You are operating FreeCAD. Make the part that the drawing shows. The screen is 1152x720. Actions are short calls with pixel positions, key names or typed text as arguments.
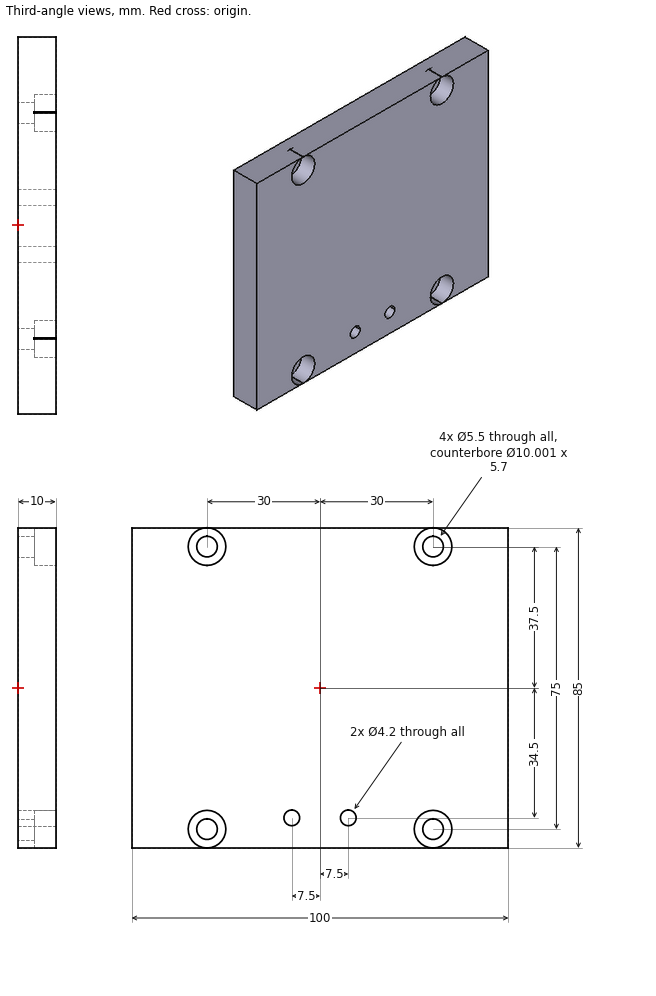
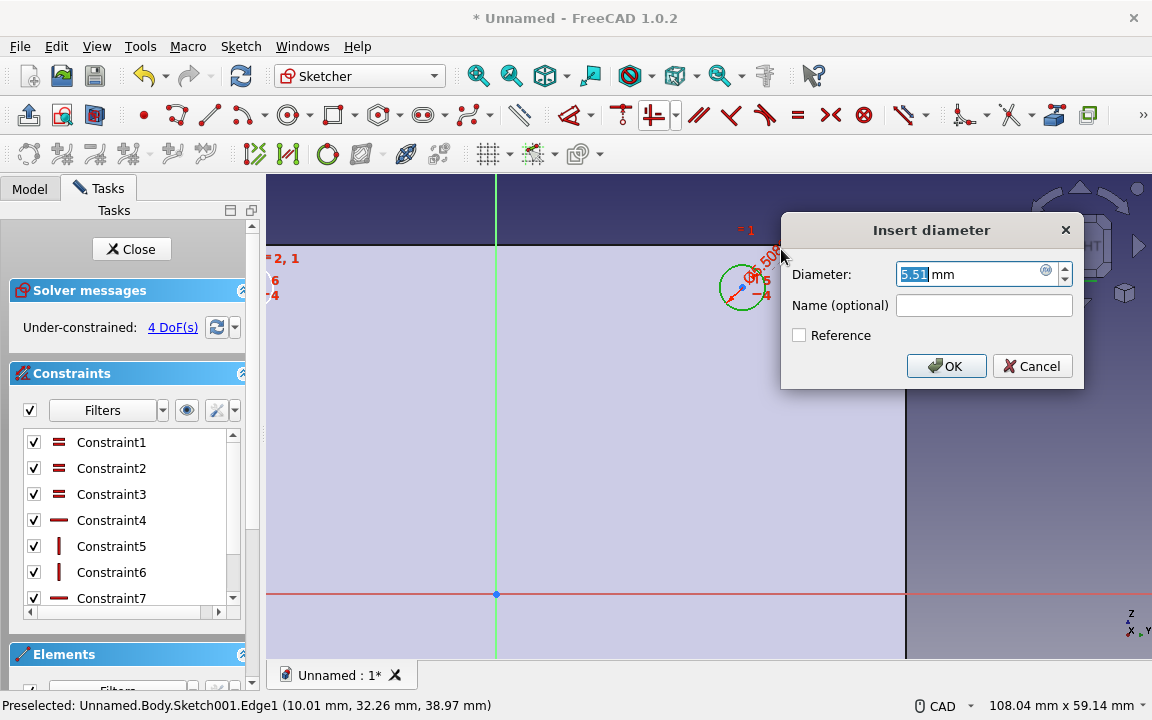
text(5.5)
key(Return)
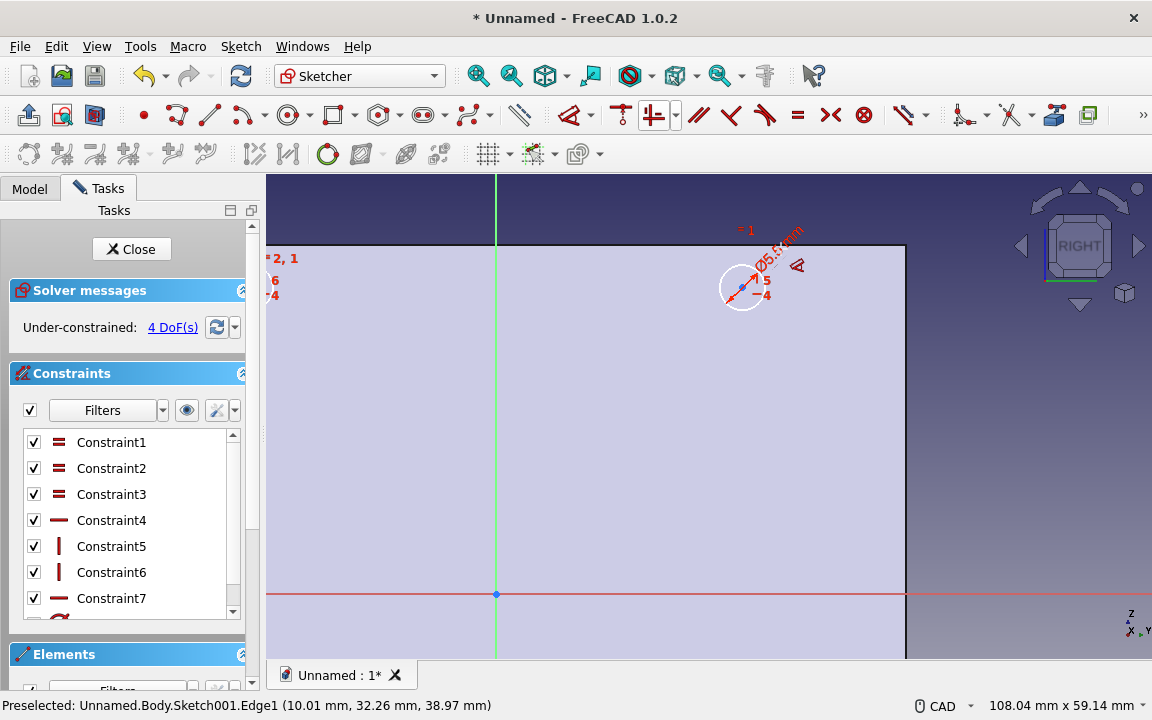
click(742, 288)
click(619, 254)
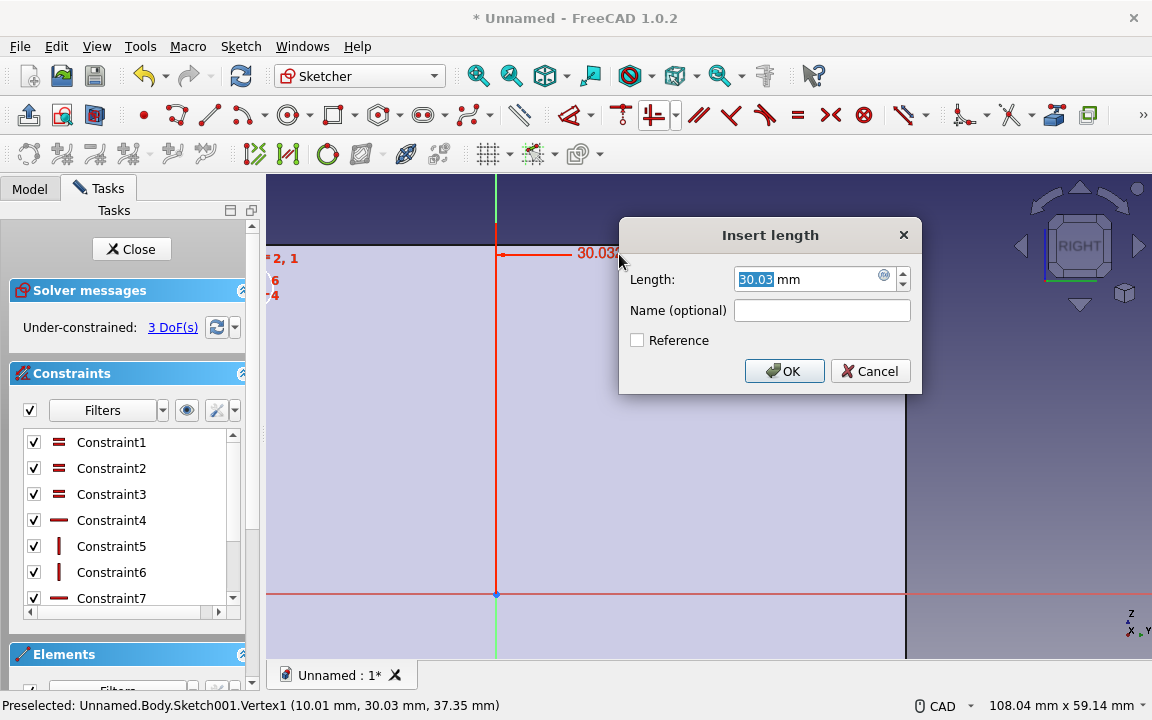
text(30)
key(Return)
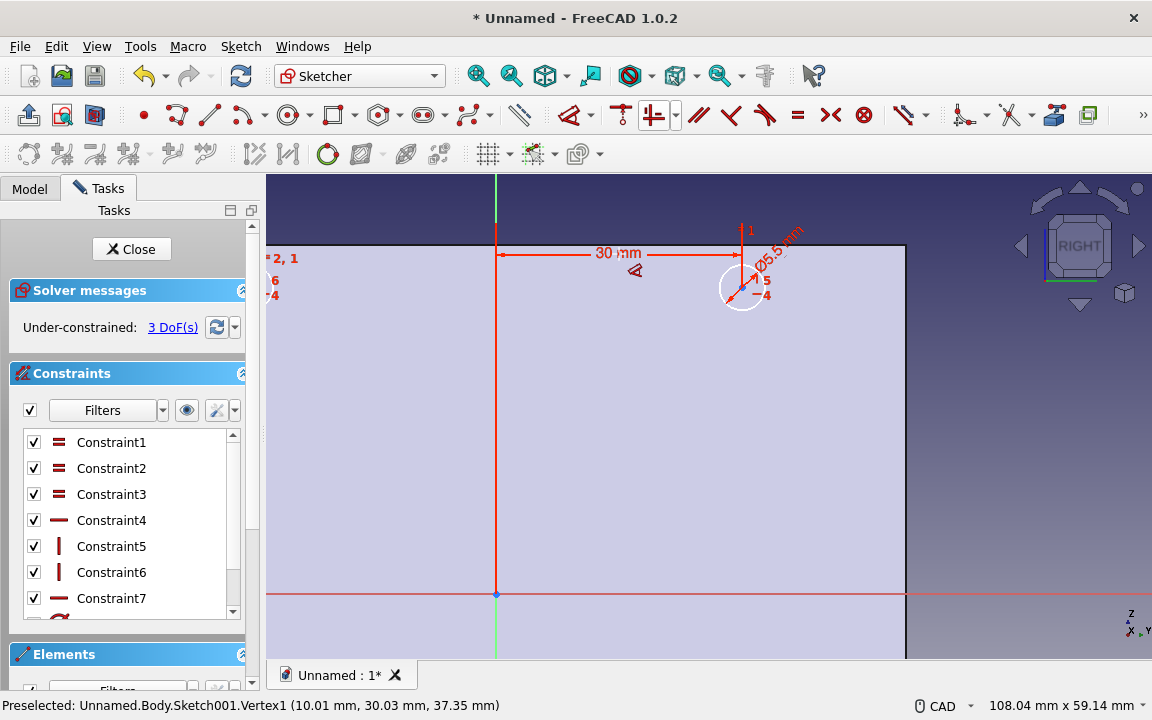
scroll(758, 272, down, 4)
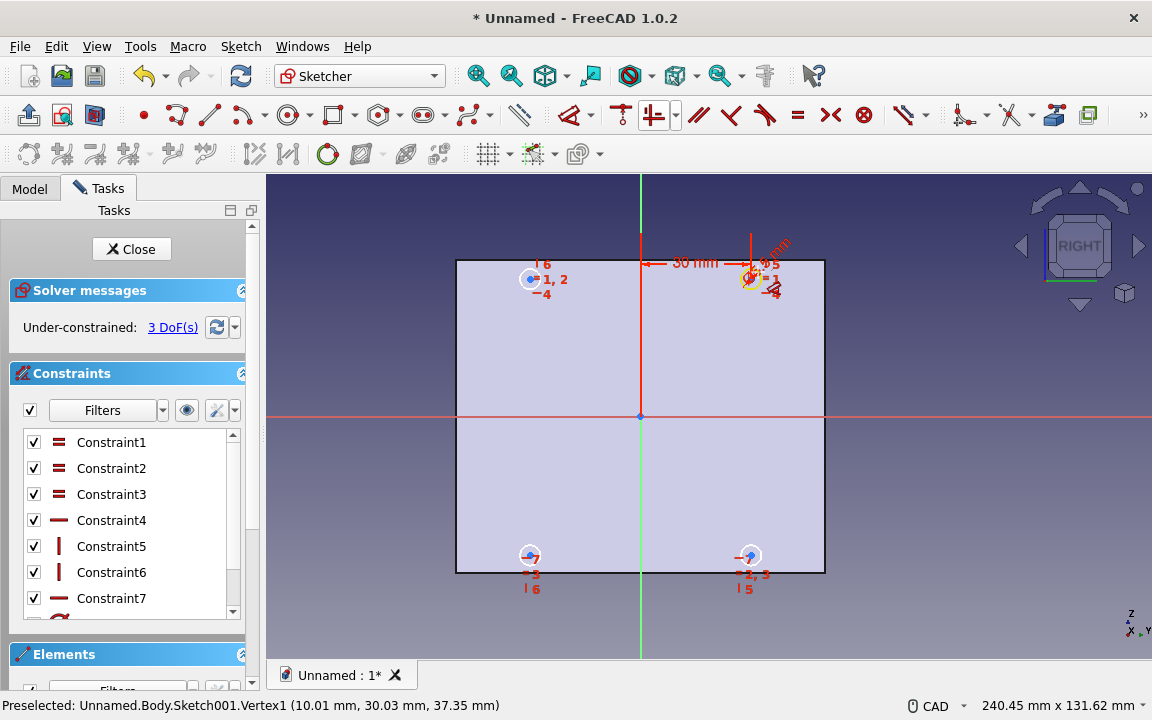
click(530, 279)
click(585, 245)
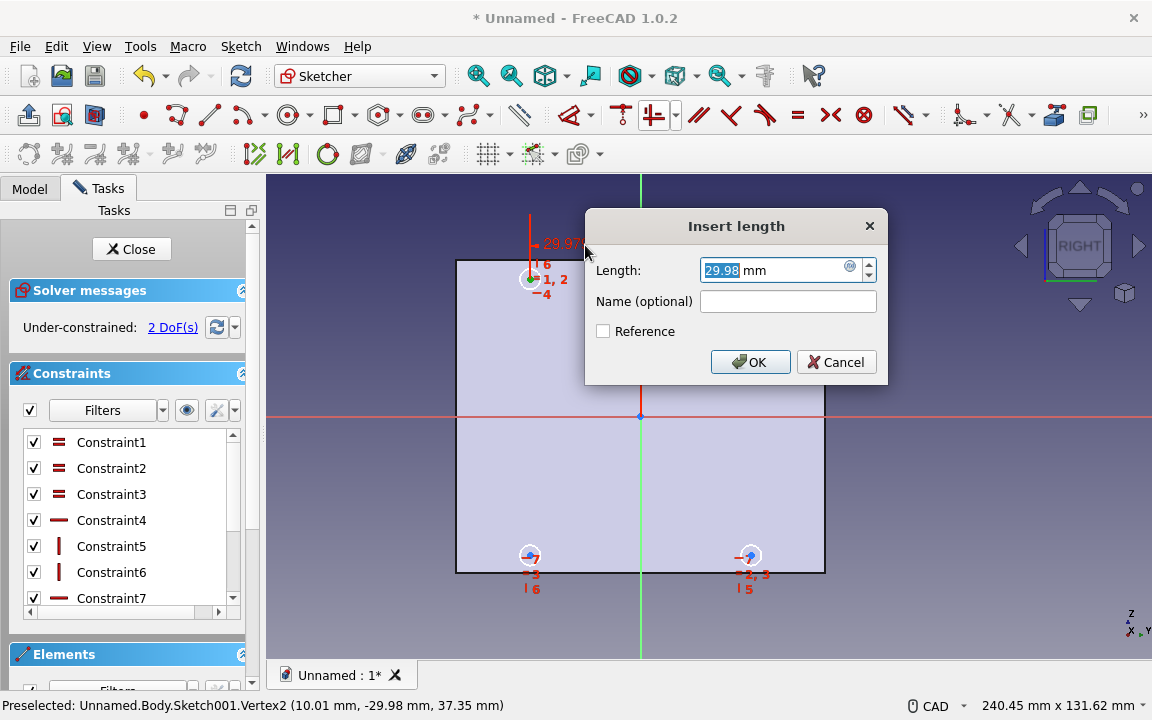
text(30)
key(Return)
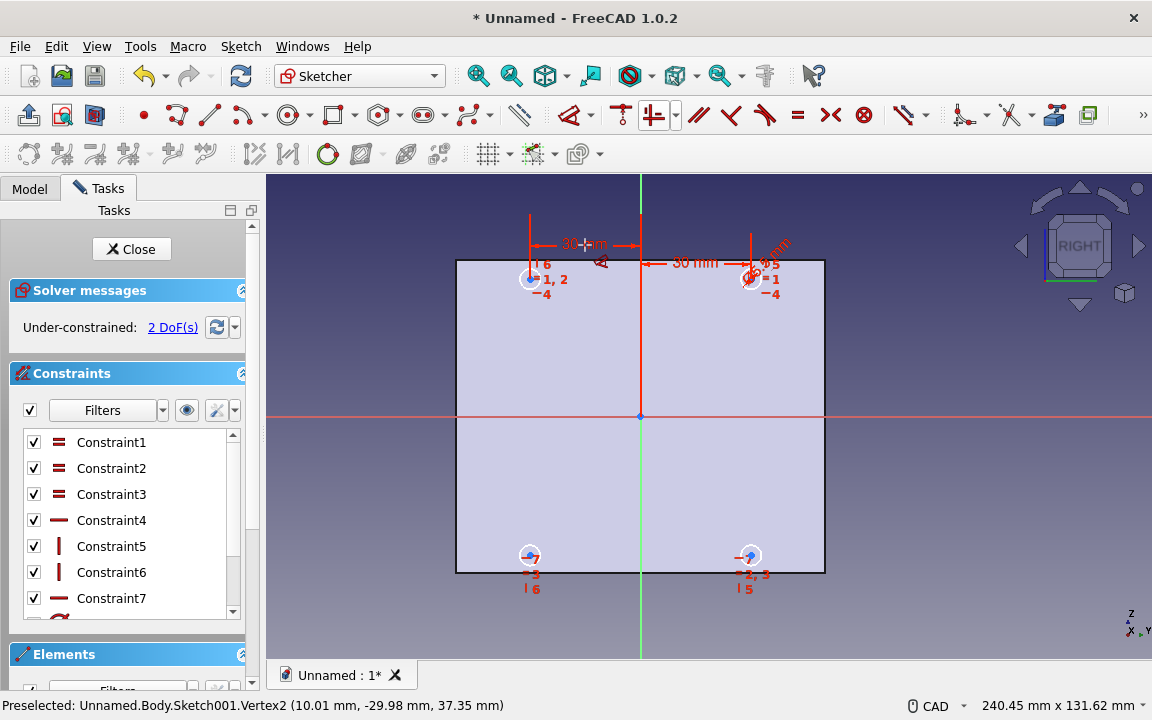
click(751, 279)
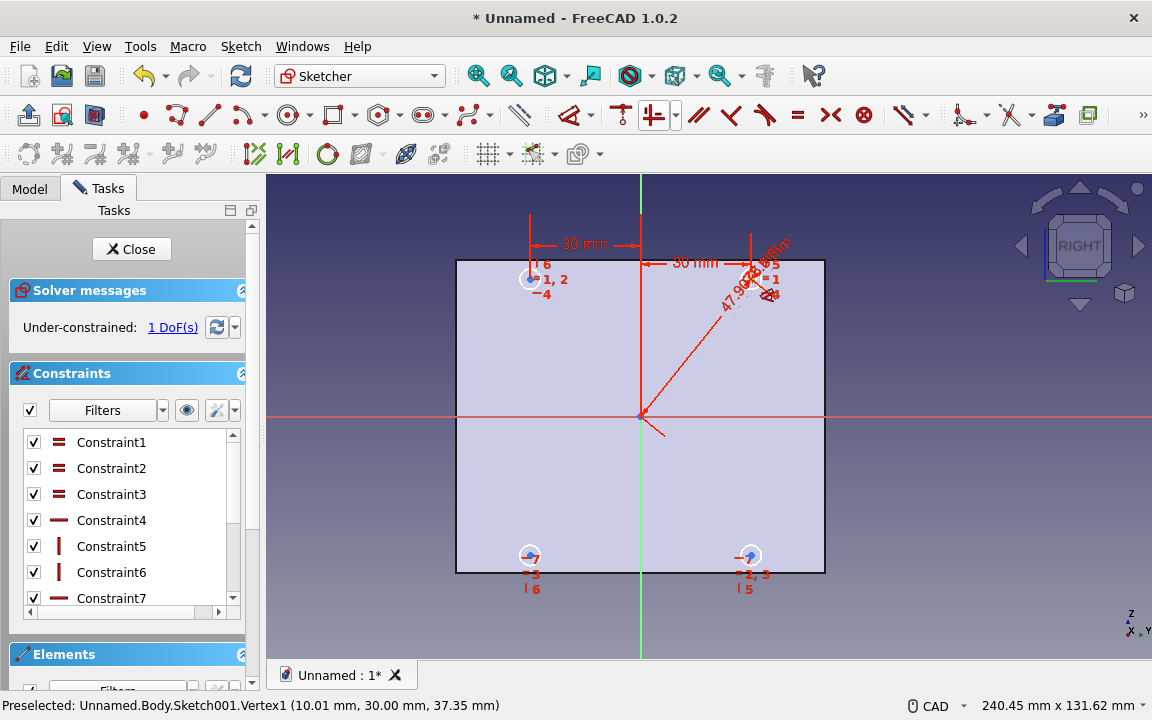
click(751, 555)
click(785, 354)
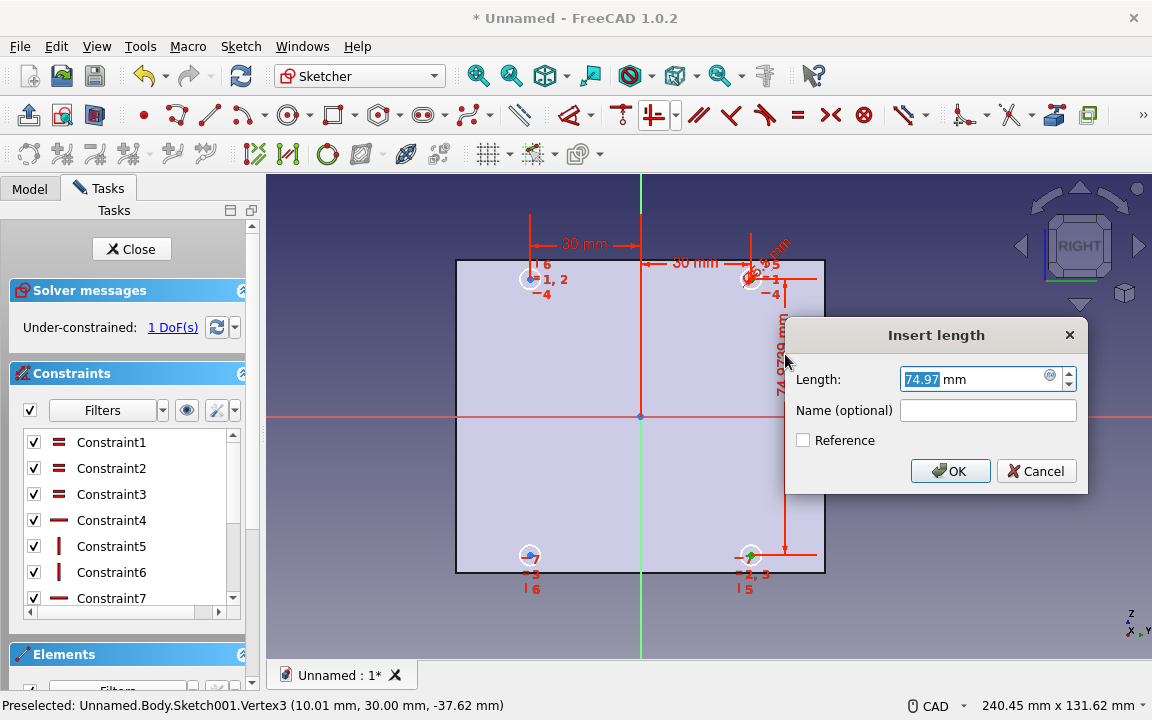
text(75)
key(Return)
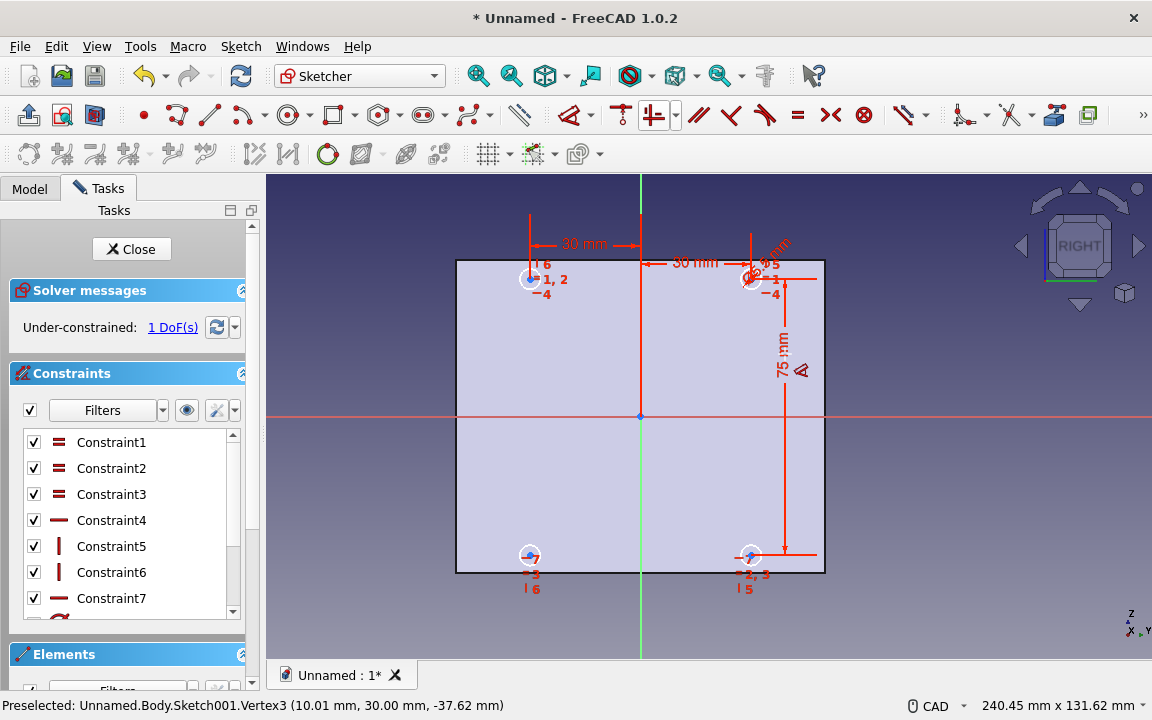
click(751, 279)
click(785, 316)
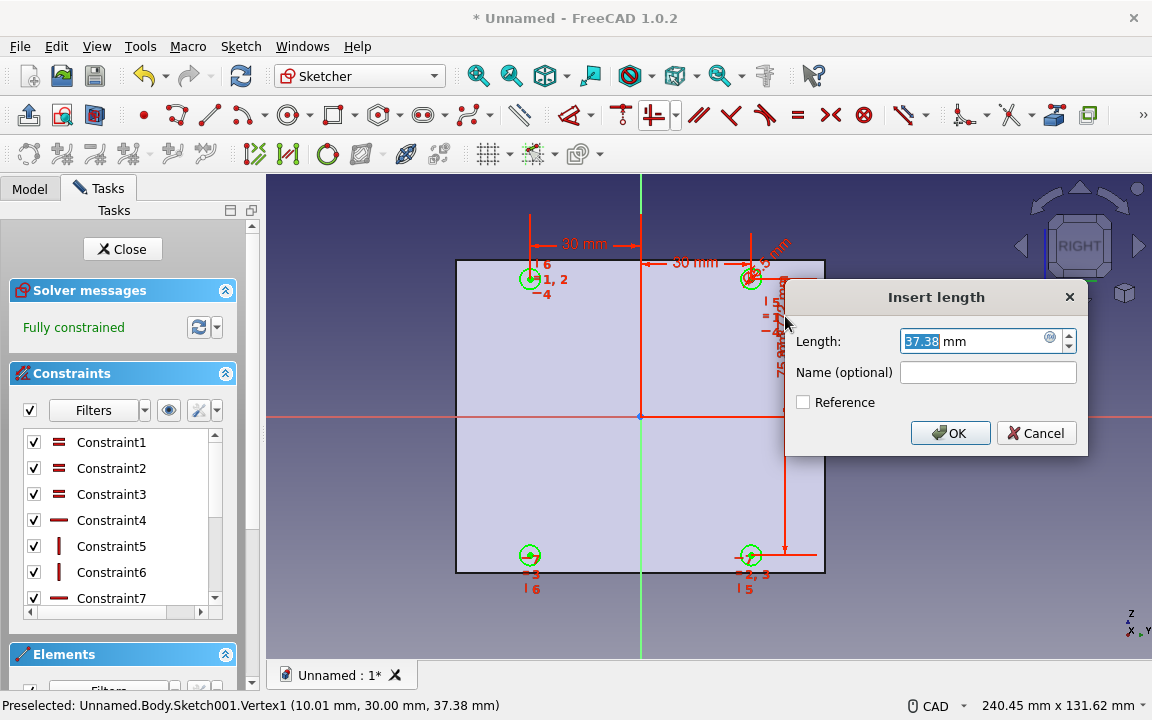
text(37.5)
key(Return)
key(Escape)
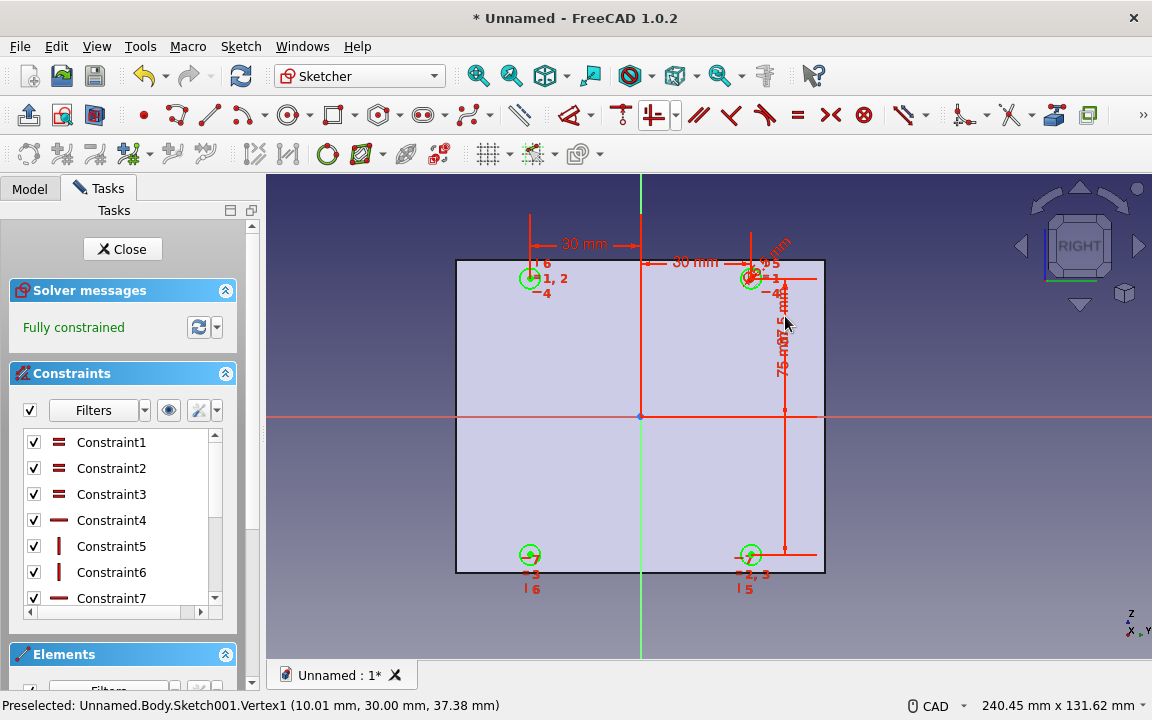
click(123, 249)